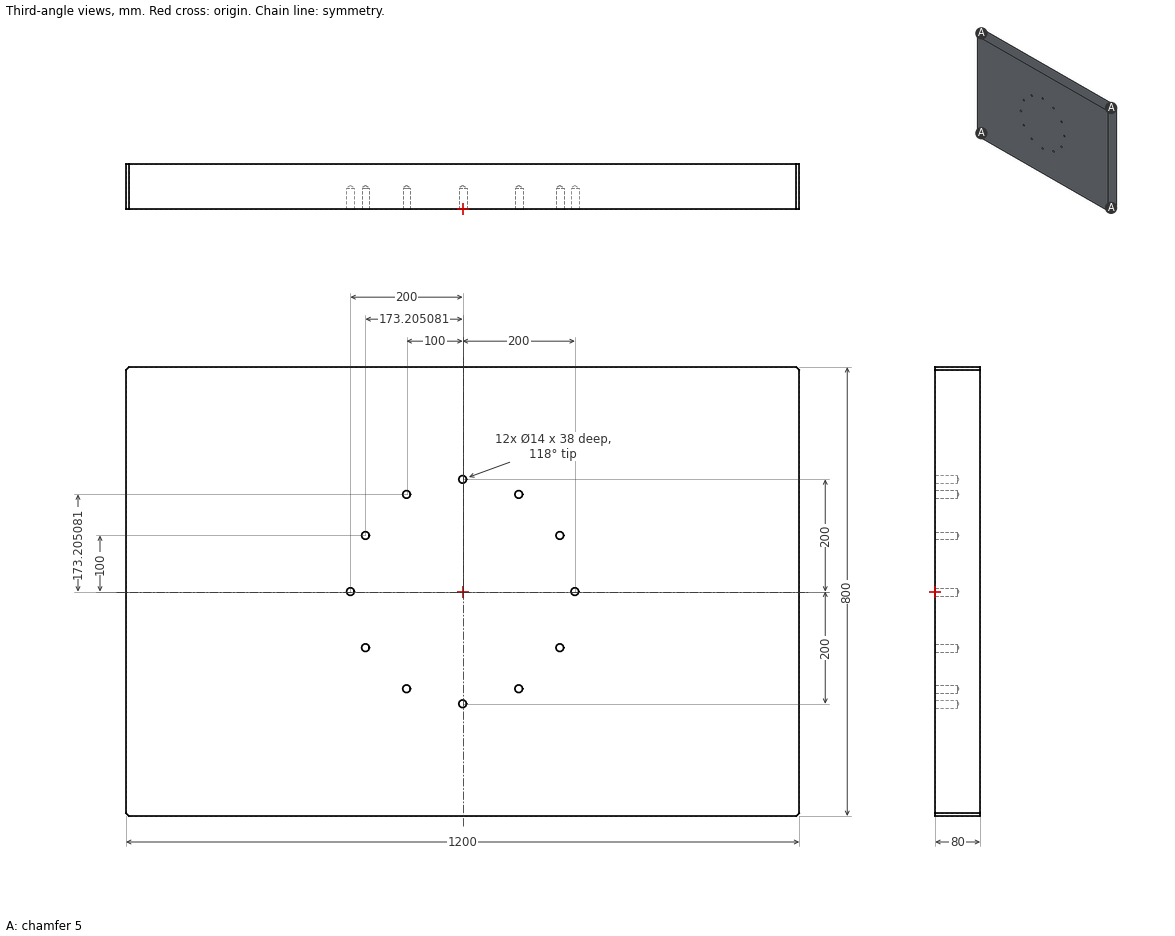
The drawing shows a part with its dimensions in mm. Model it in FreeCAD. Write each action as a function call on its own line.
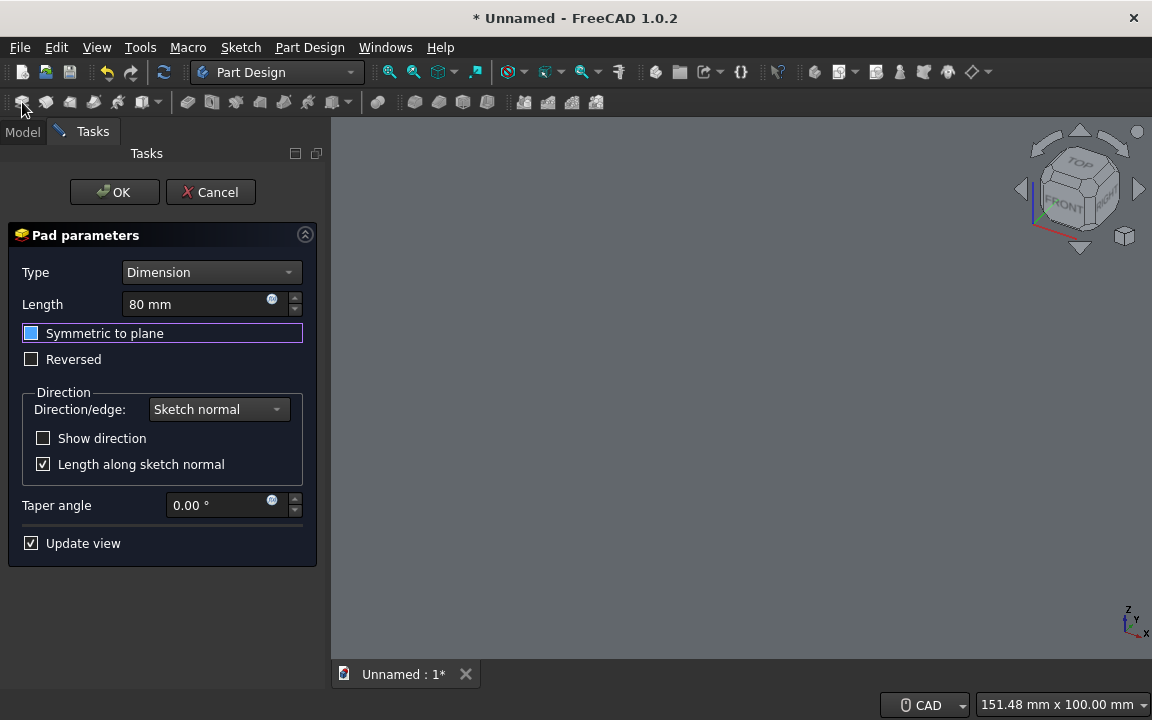
click(30, 359)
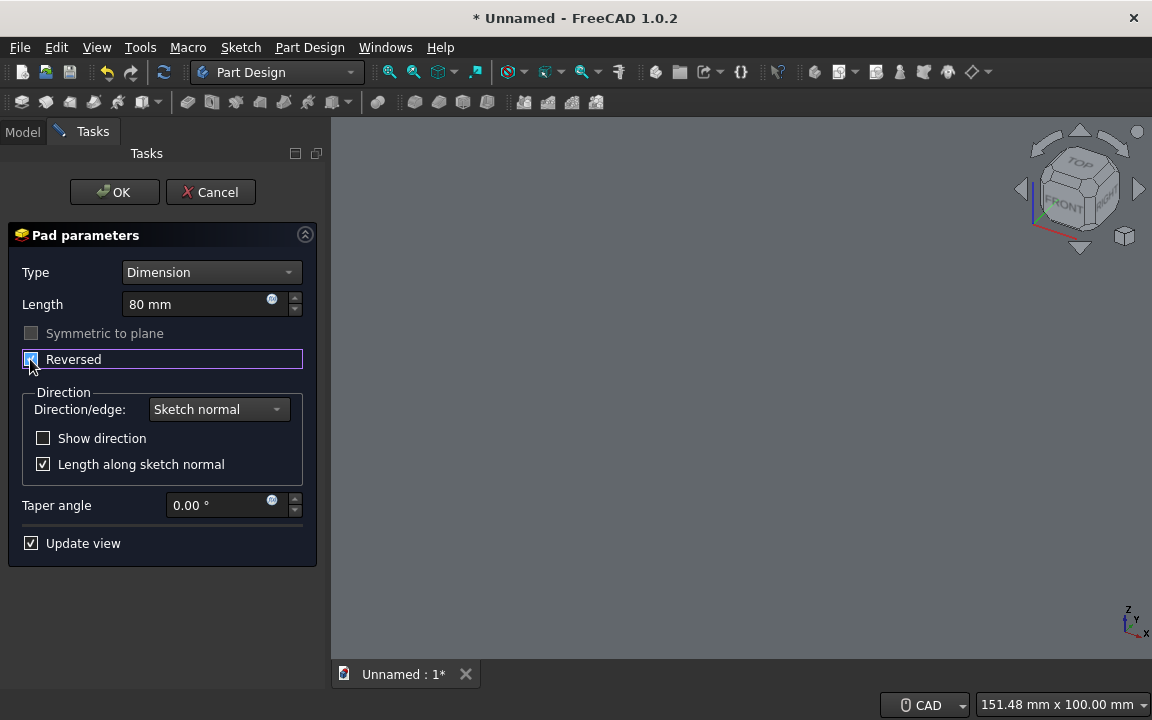
click(115, 192)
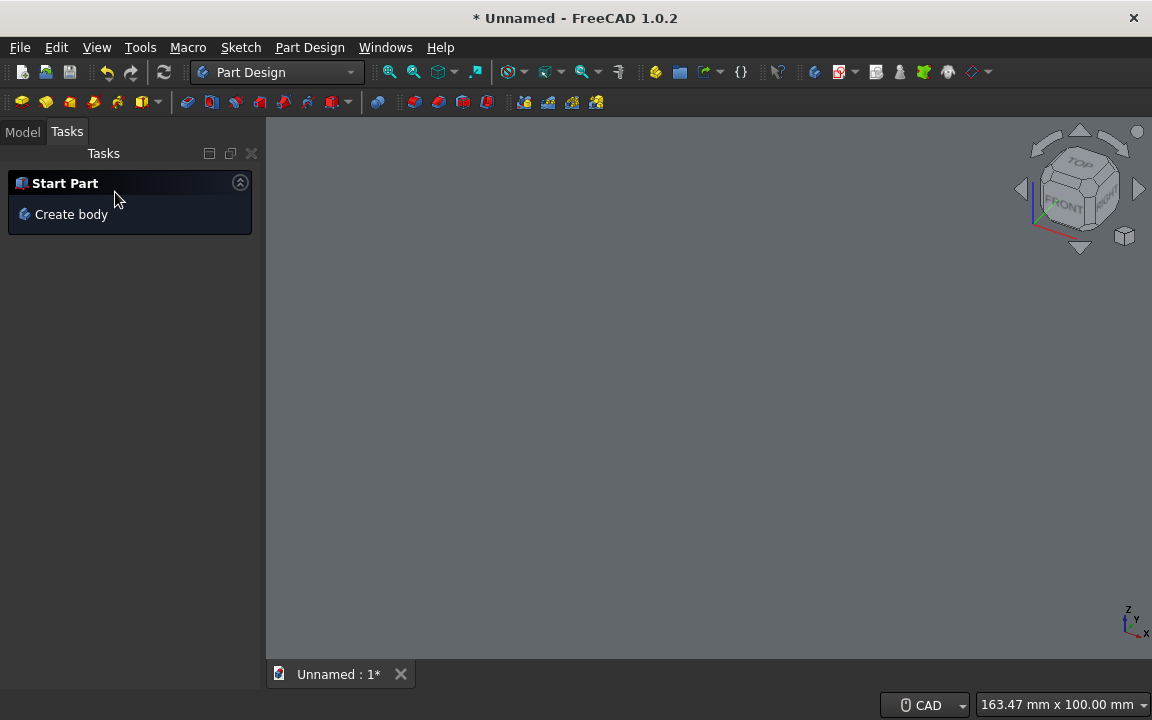
click(390, 72)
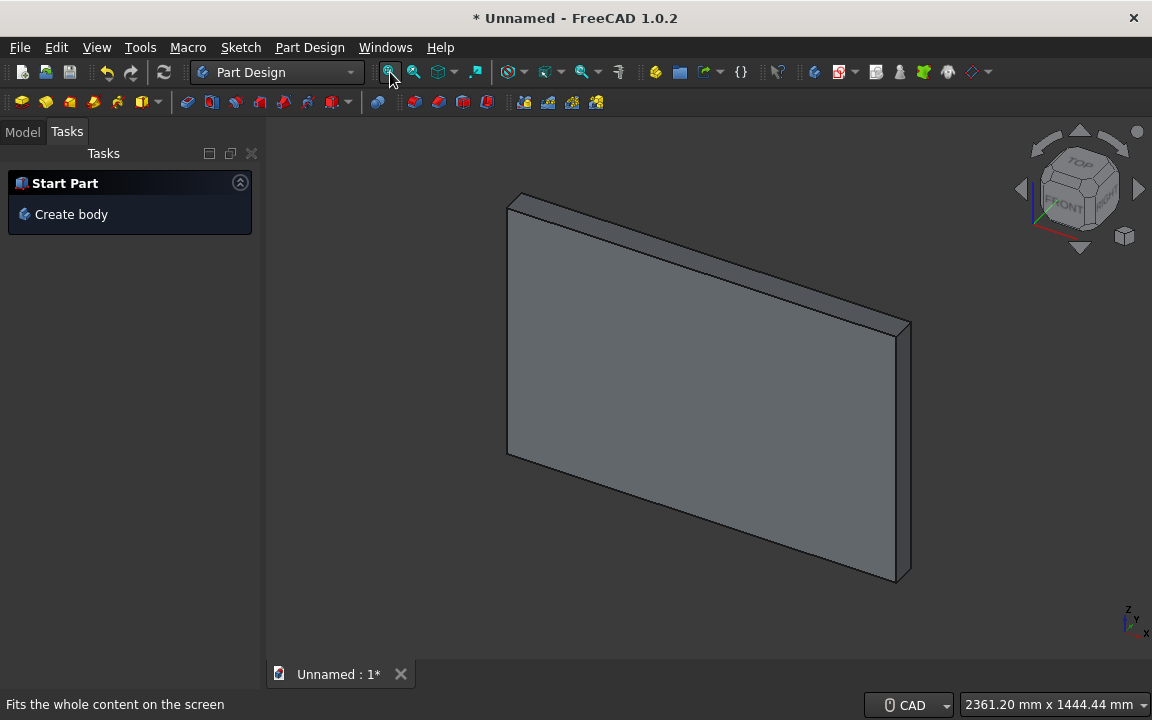
click(904, 329)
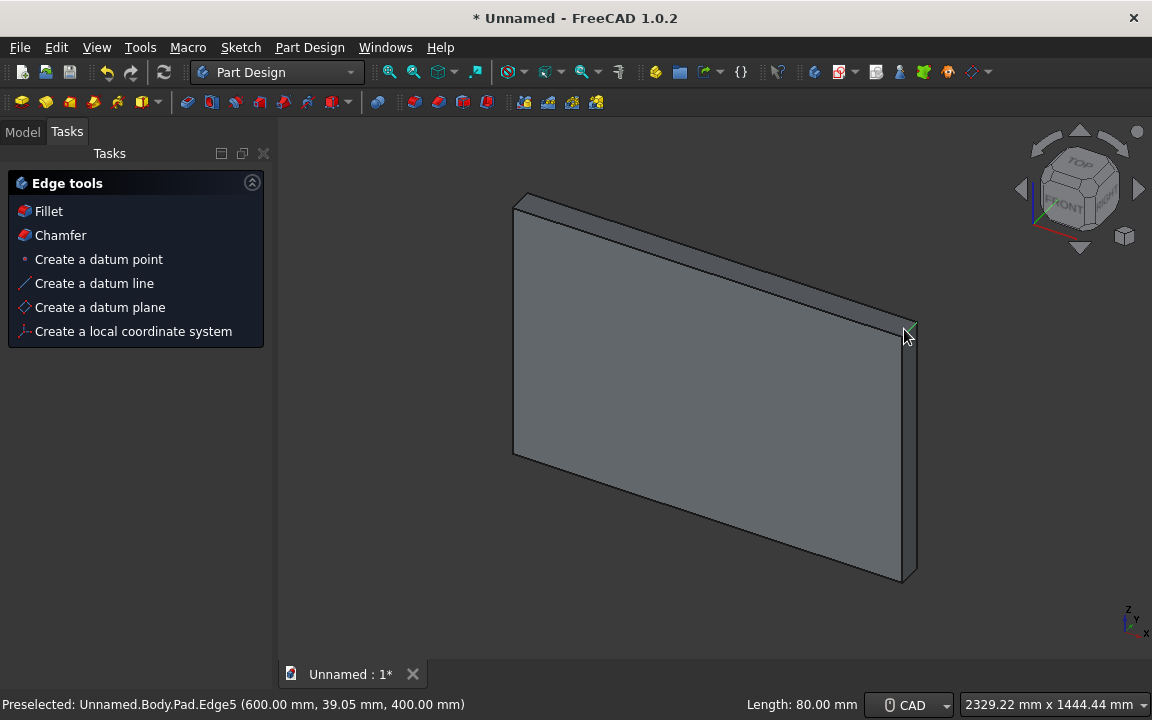
key(0)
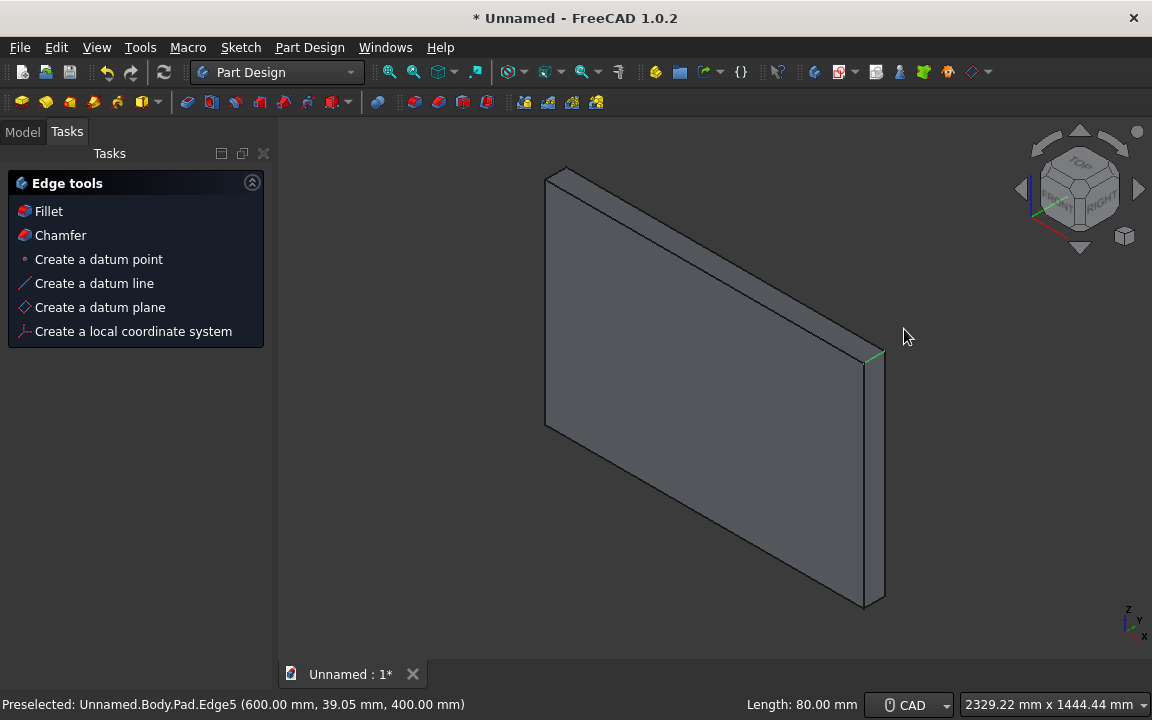
key(2)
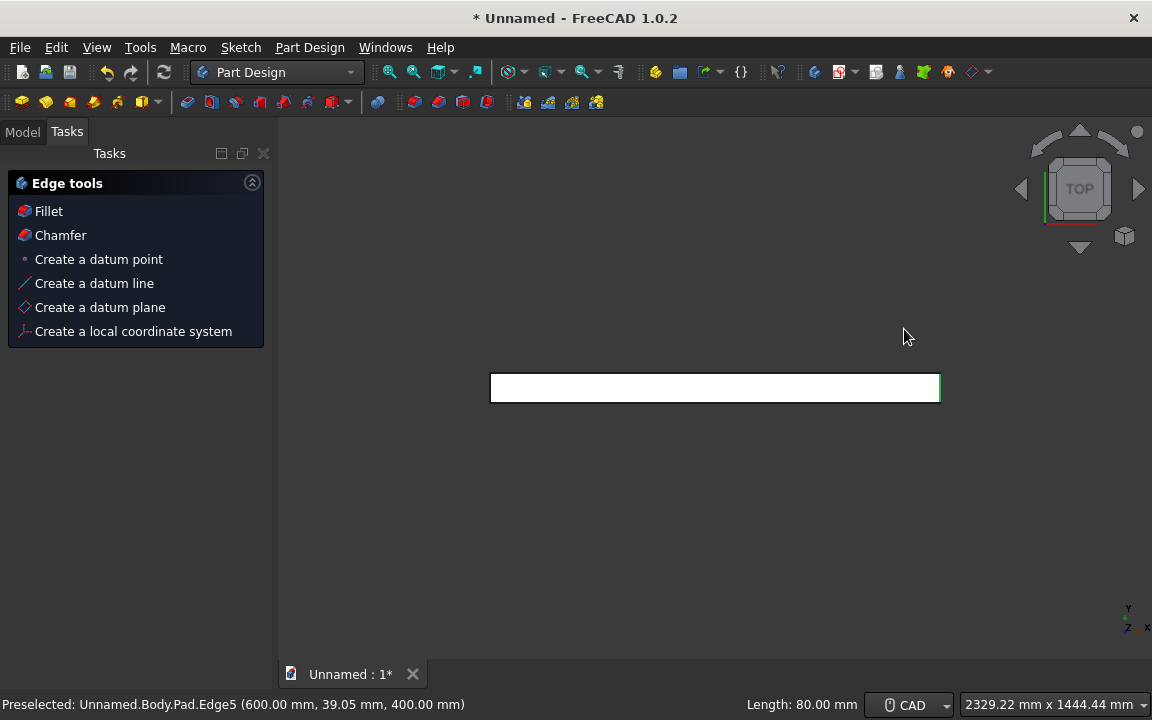
click(490, 387, ctrl)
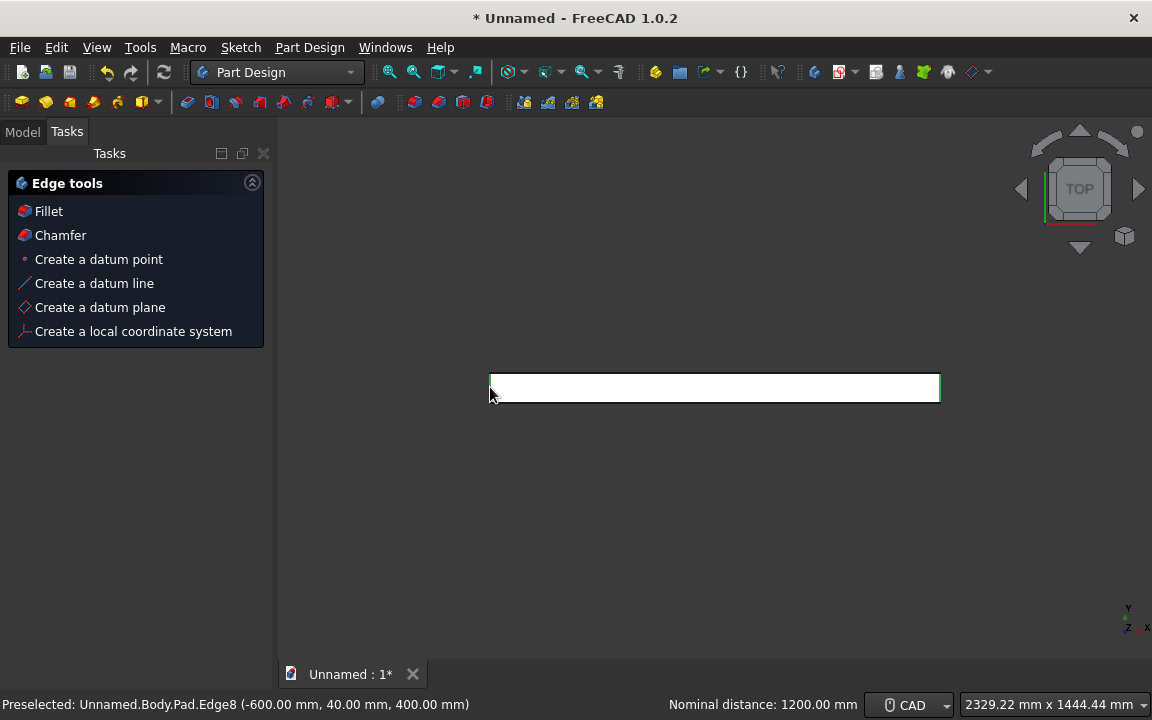
key(1)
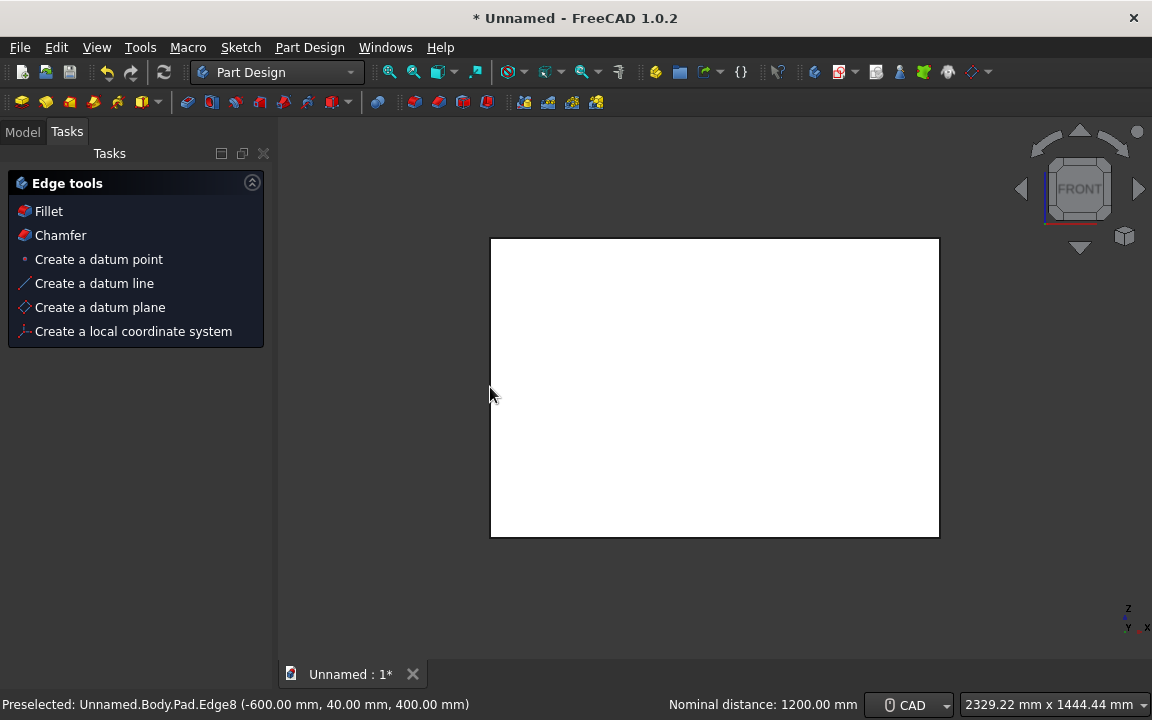
key(3)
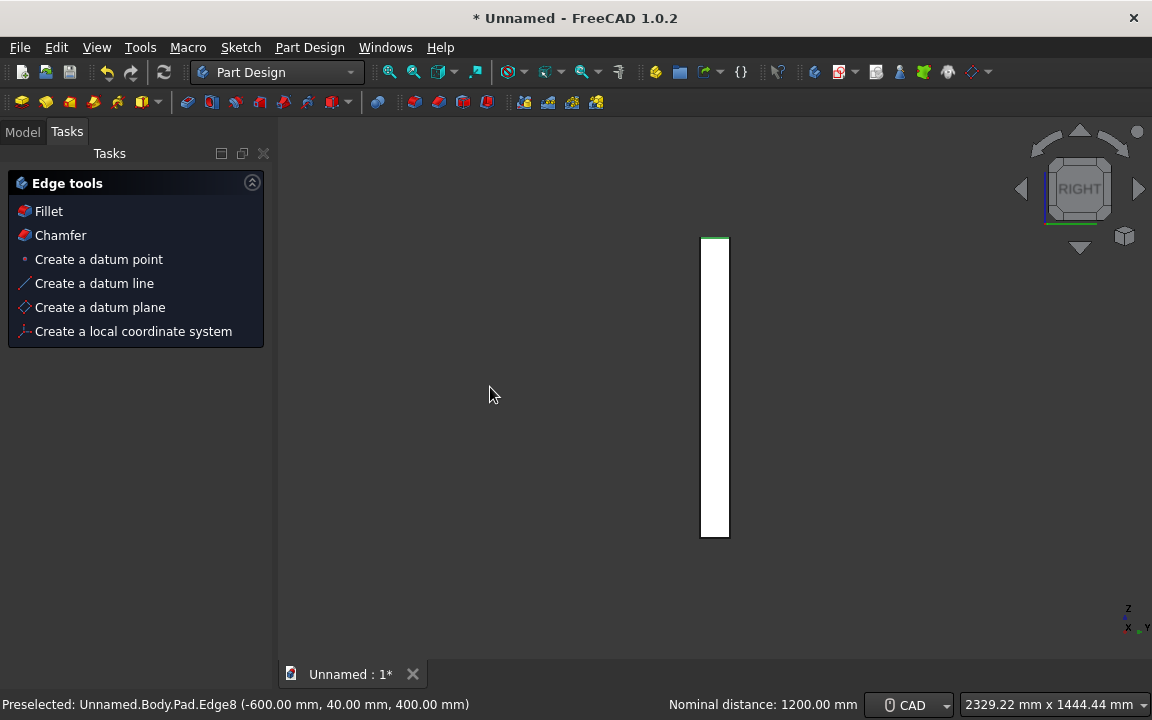
click(715, 537, ctrl)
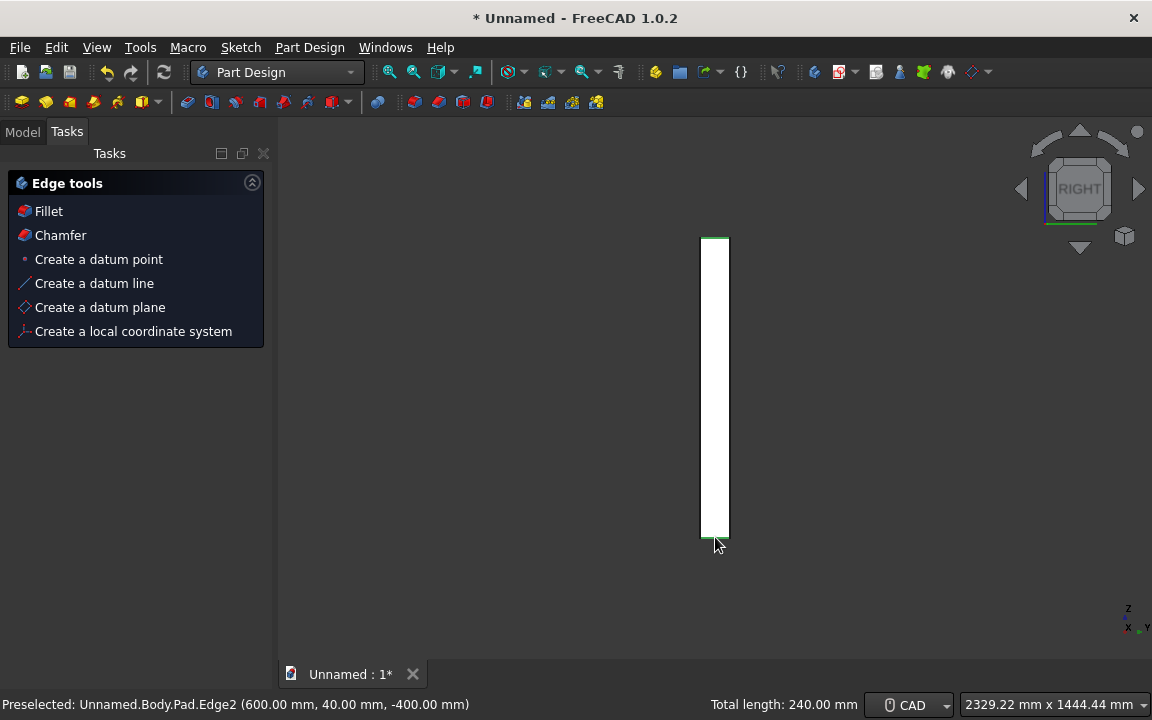
key(5)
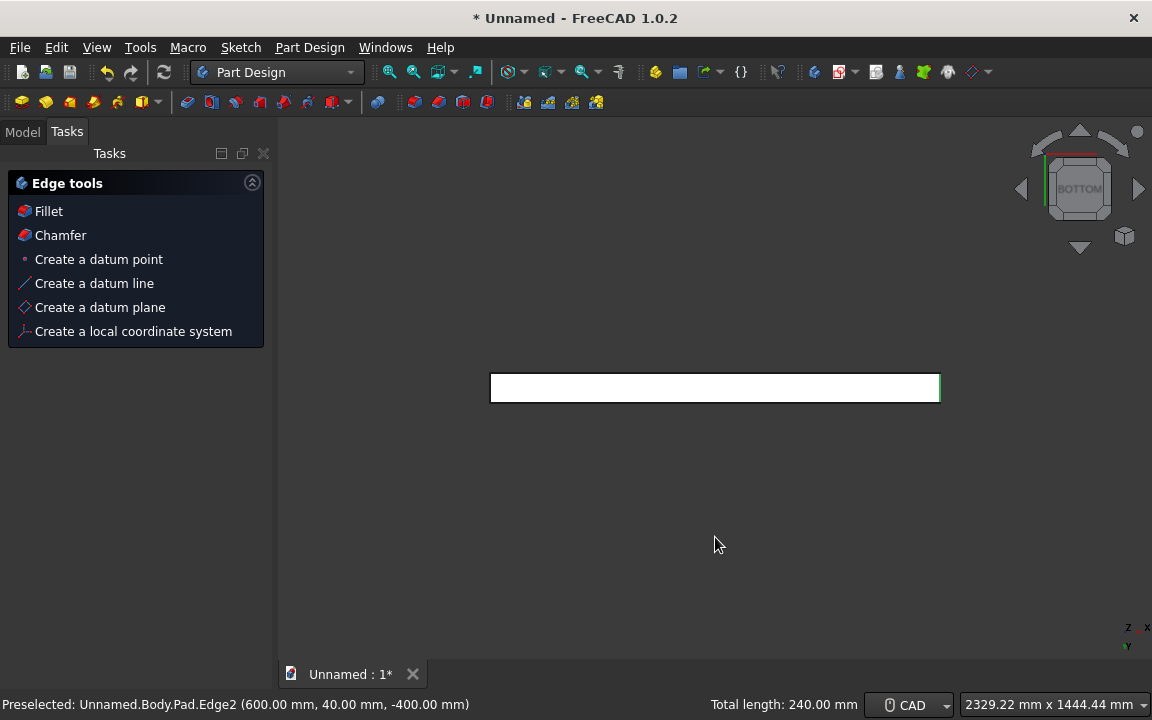
click(490, 387, ctrl)